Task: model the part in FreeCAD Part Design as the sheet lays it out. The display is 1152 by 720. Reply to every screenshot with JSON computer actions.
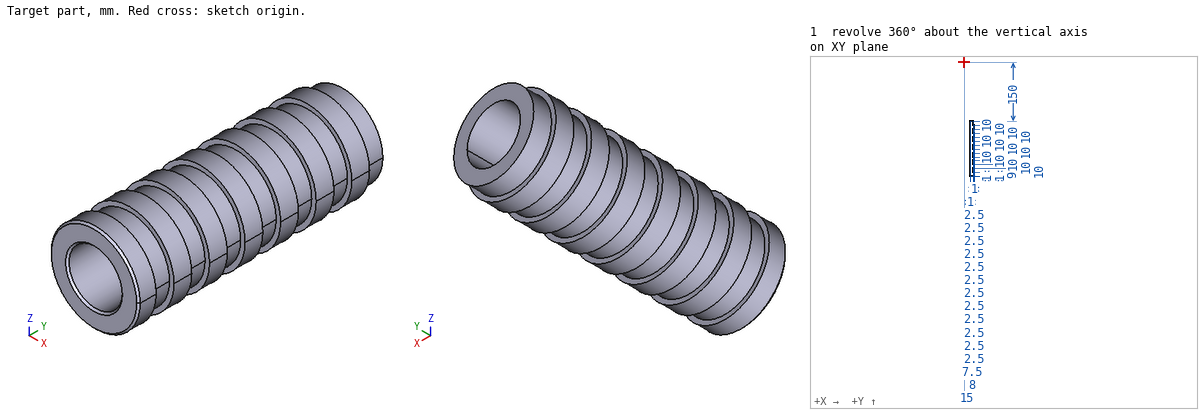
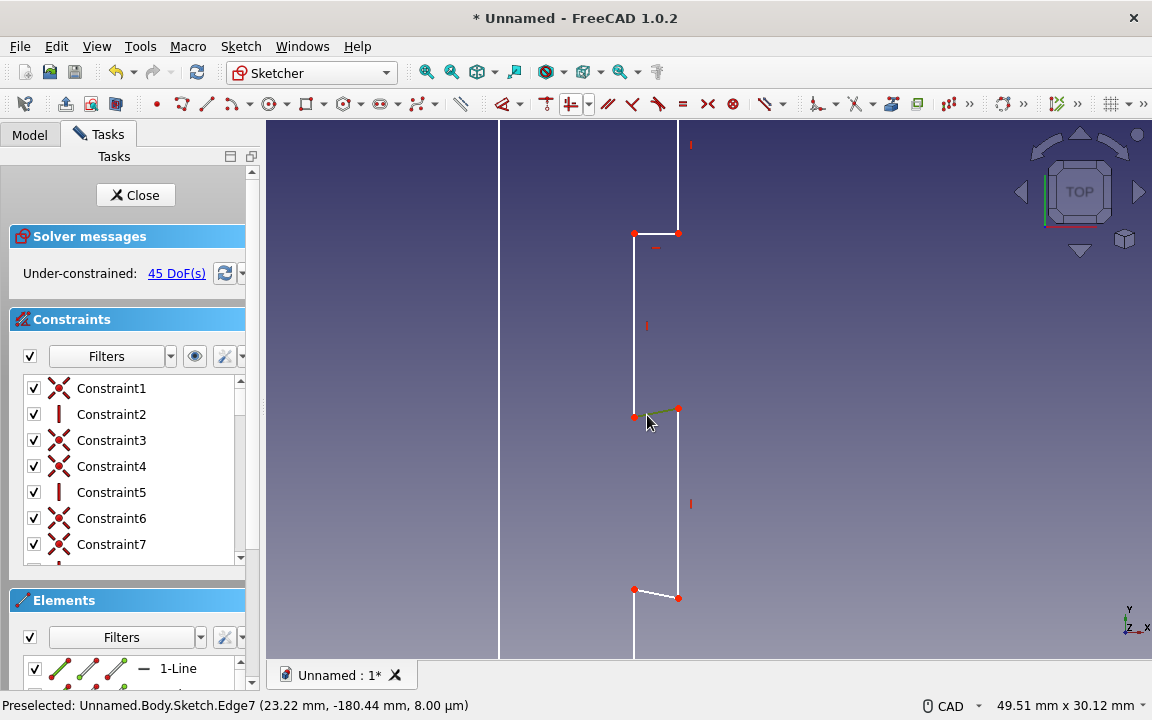
{"action": "key", "text": "h"}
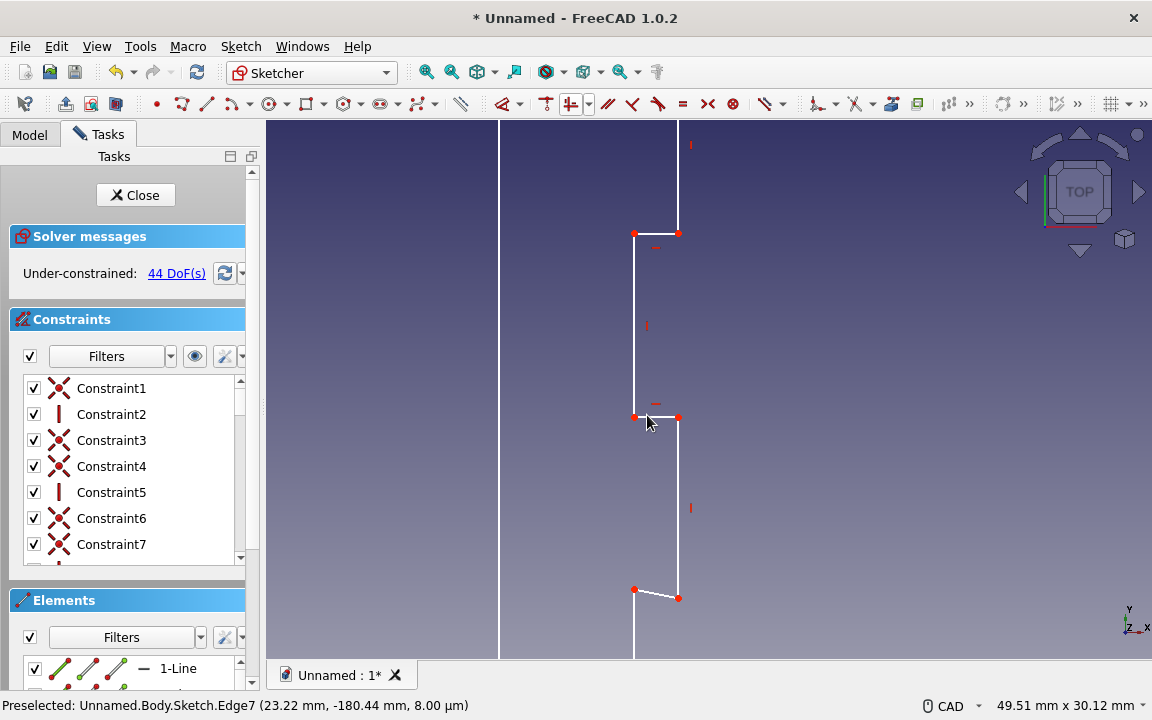
{"action": "left_click", "coordinate": [665, 596]}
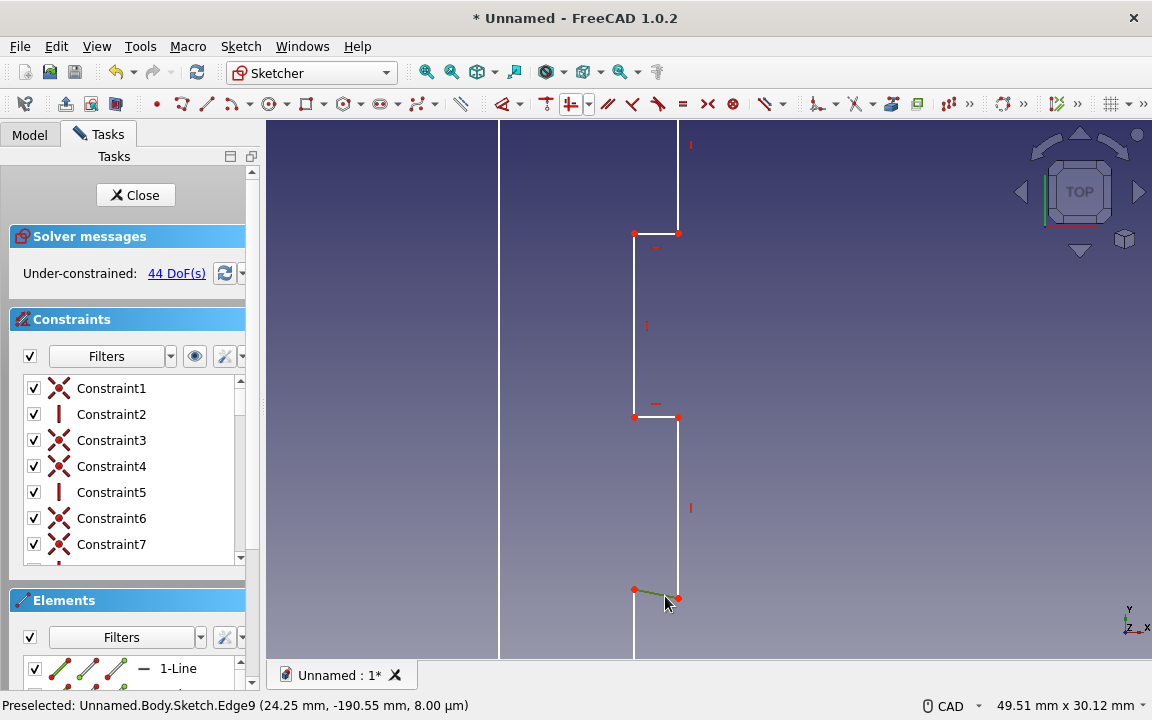
{"action": "left_click", "coordinate": [588, 104]}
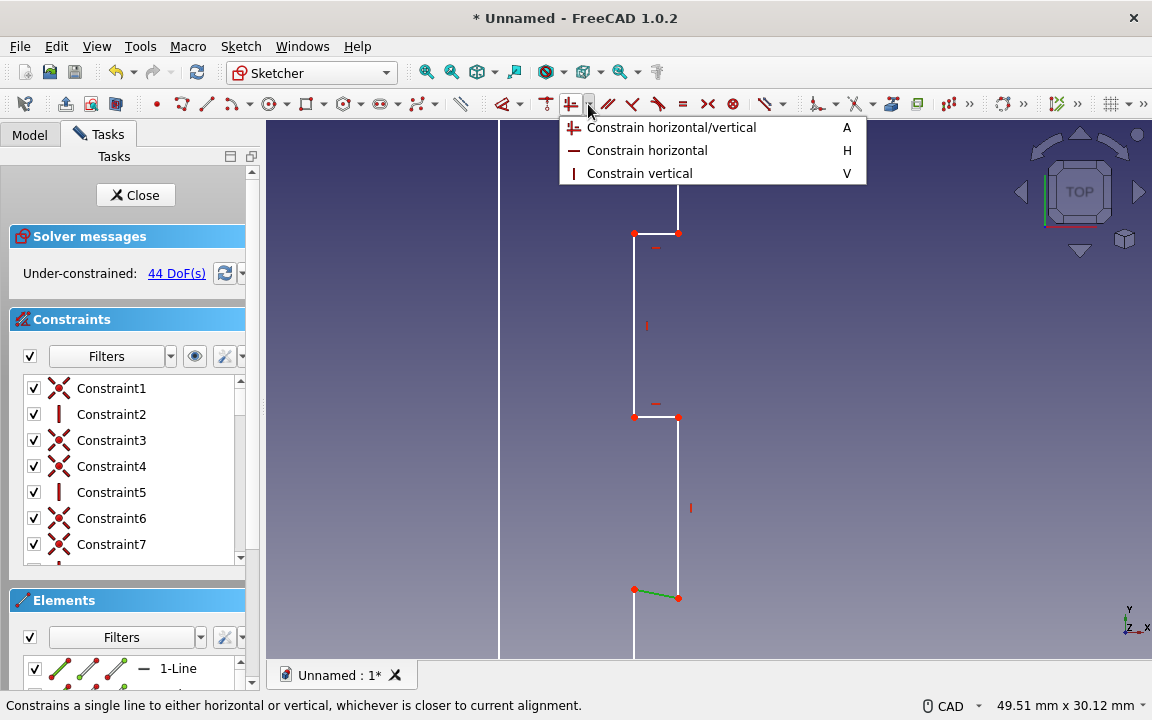
{"action": "left_click", "coordinate": [713, 150]}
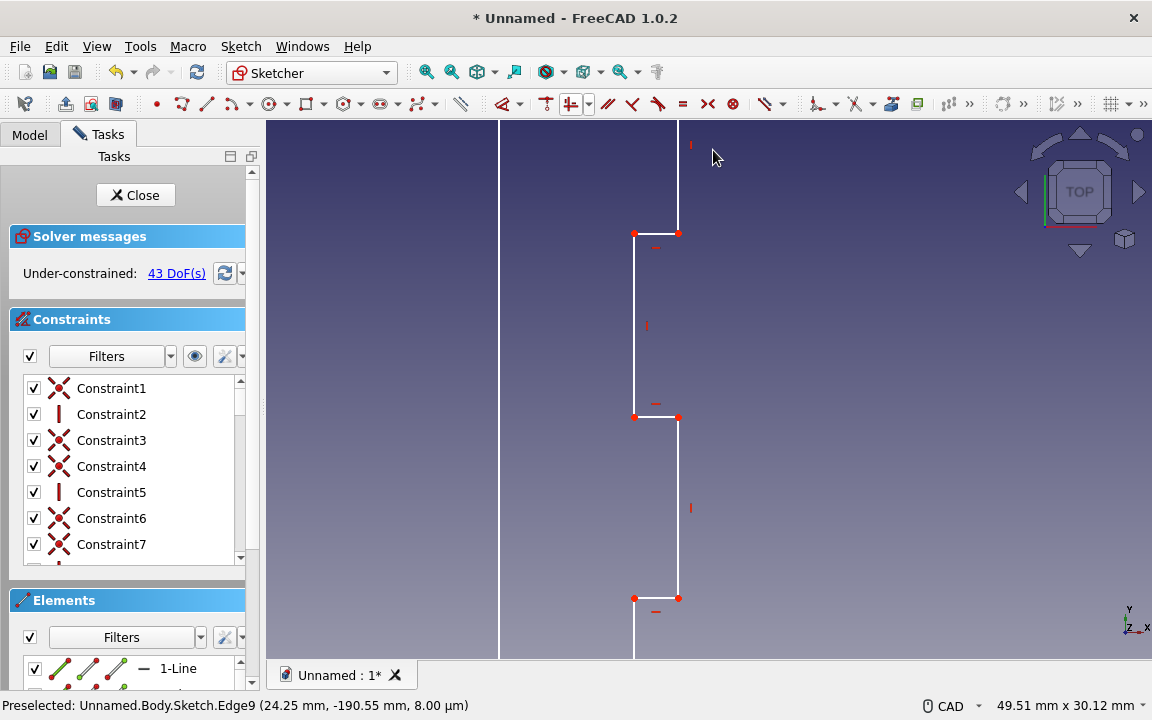
{"action": "scroll", "coordinate": [653, 429], "scroll_direction": "down", "scroll_amount": 14}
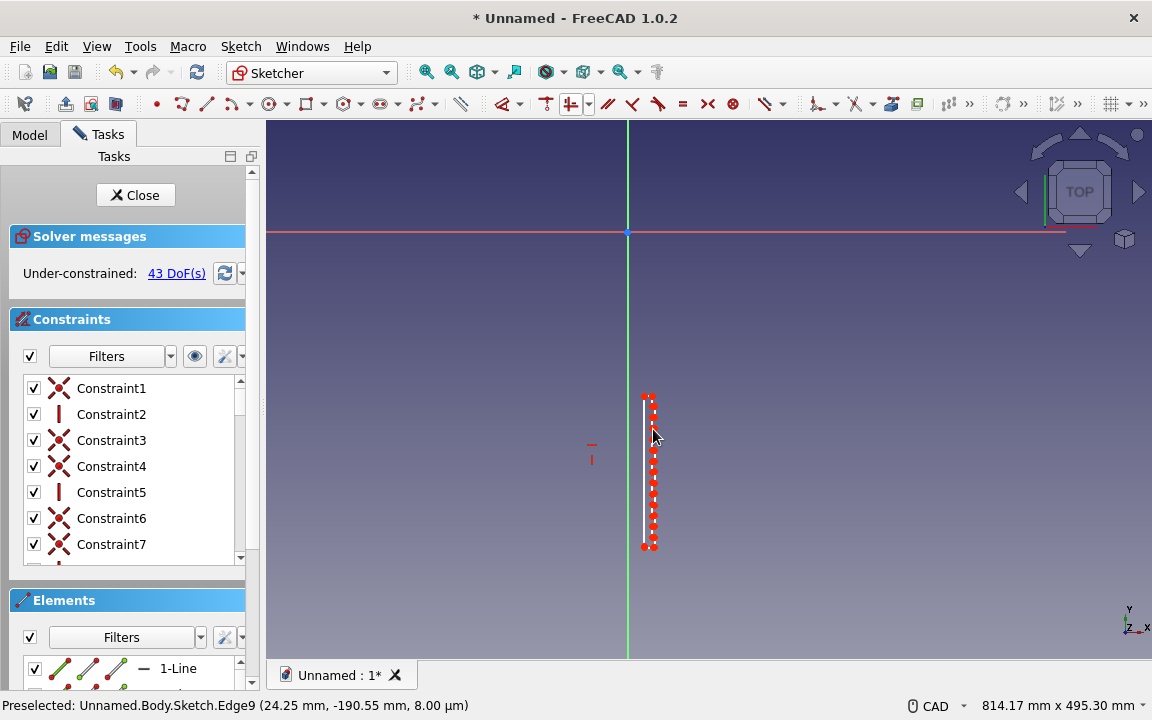
{"action": "scroll", "coordinate": [653, 451], "scroll_direction": "up", "scroll_amount": 14}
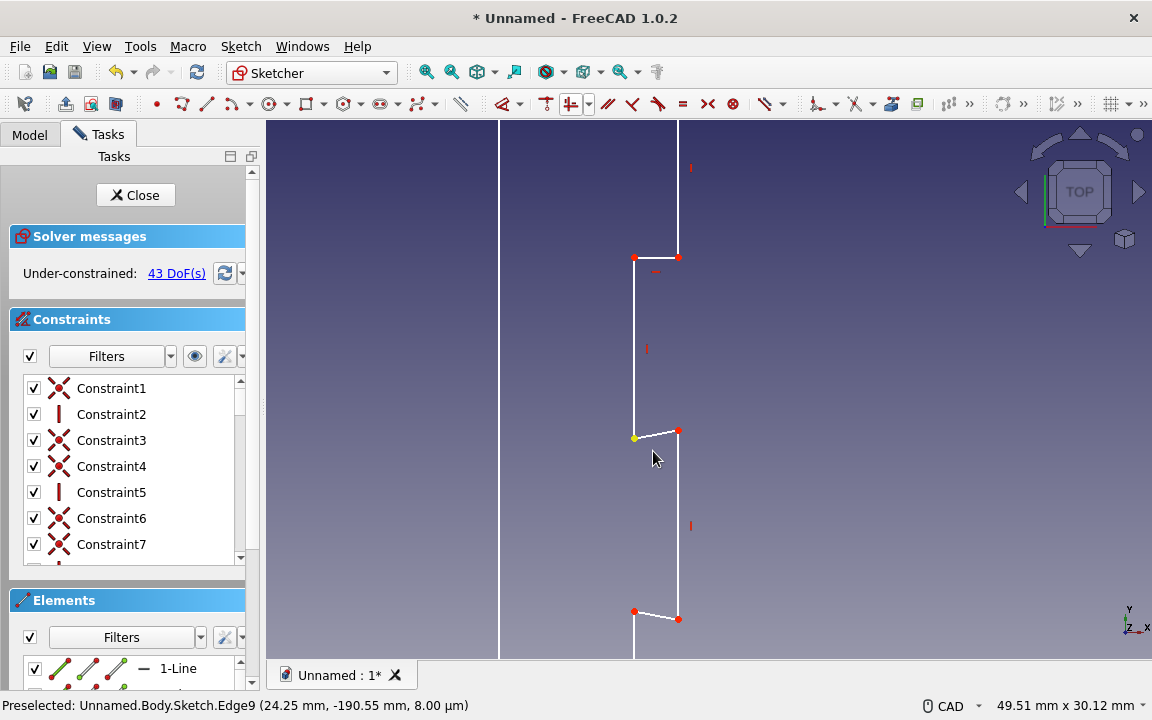
{"action": "left_click", "coordinate": [647, 436]}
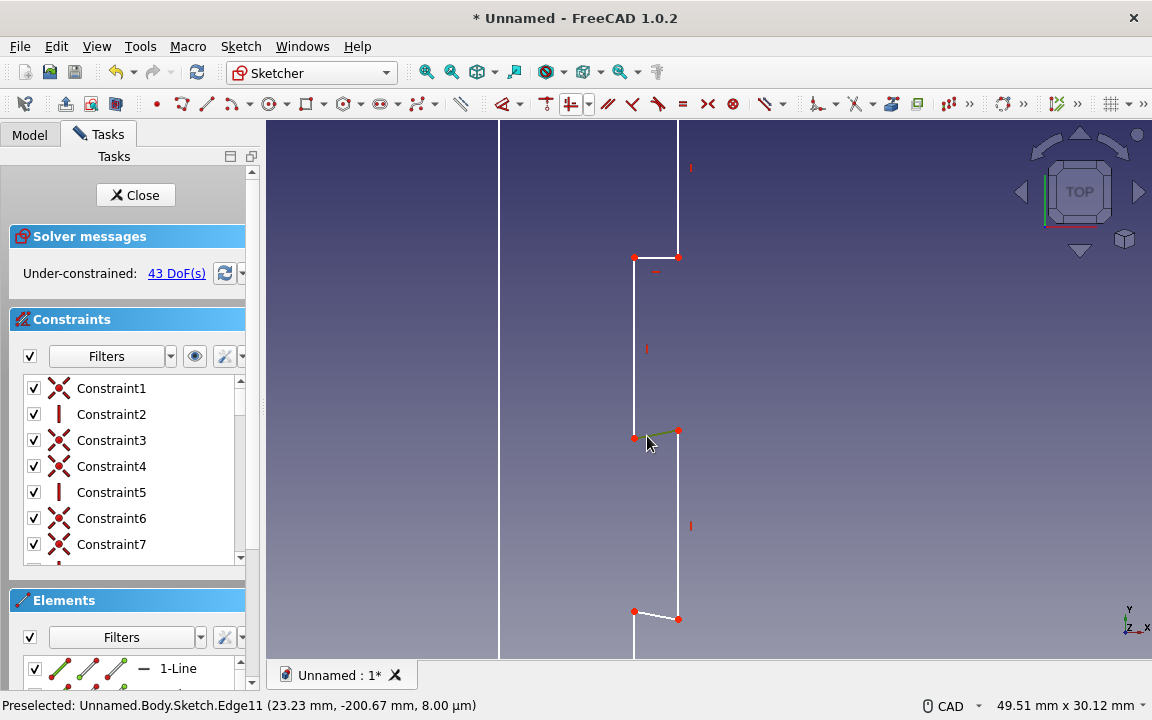
{"action": "key", "text": "h"}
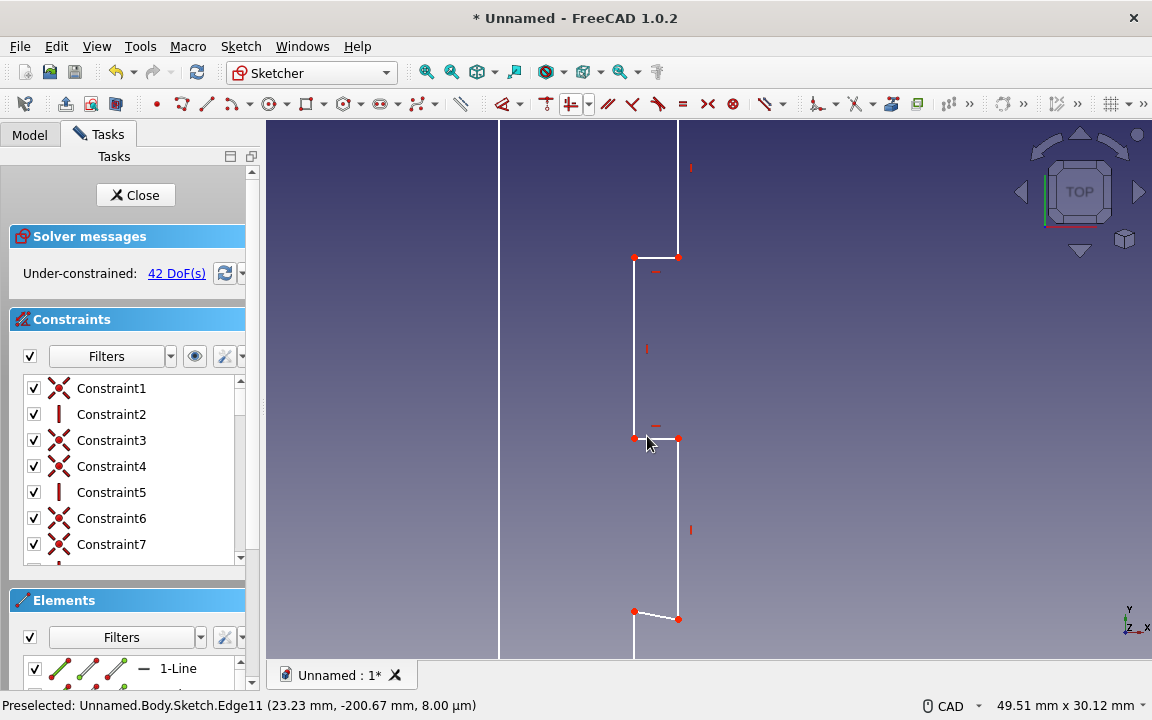
{"action": "left_click", "coordinate": [665, 617]}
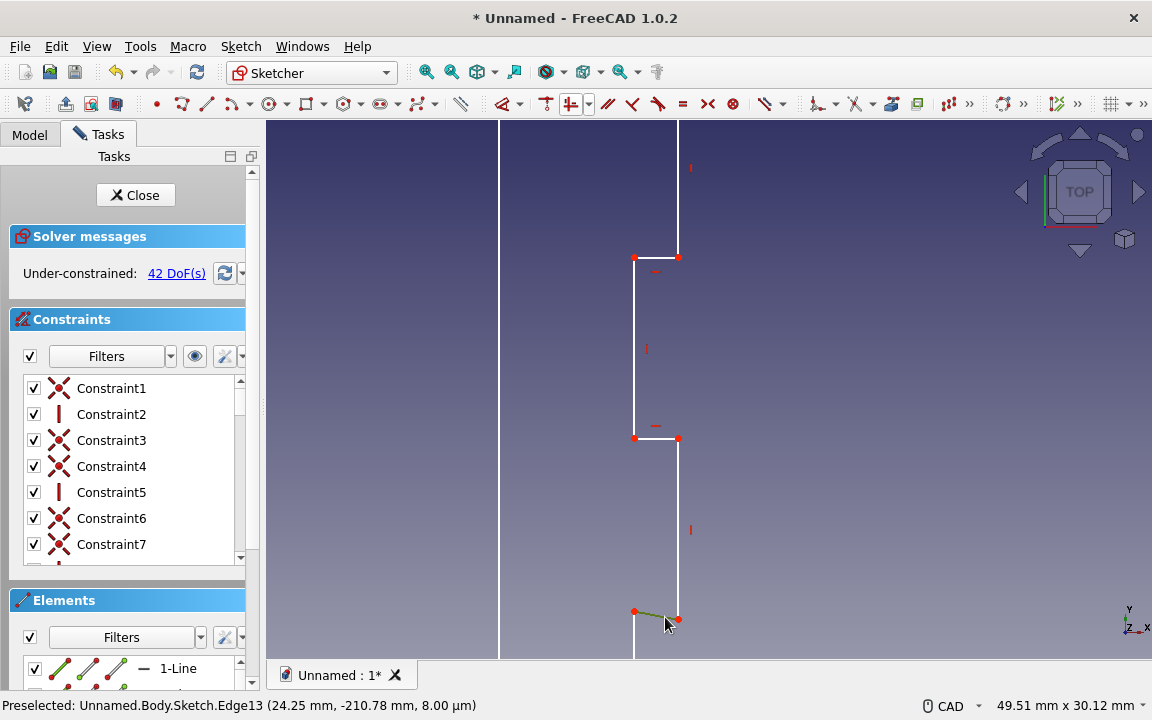
{"action": "key", "text": "h"}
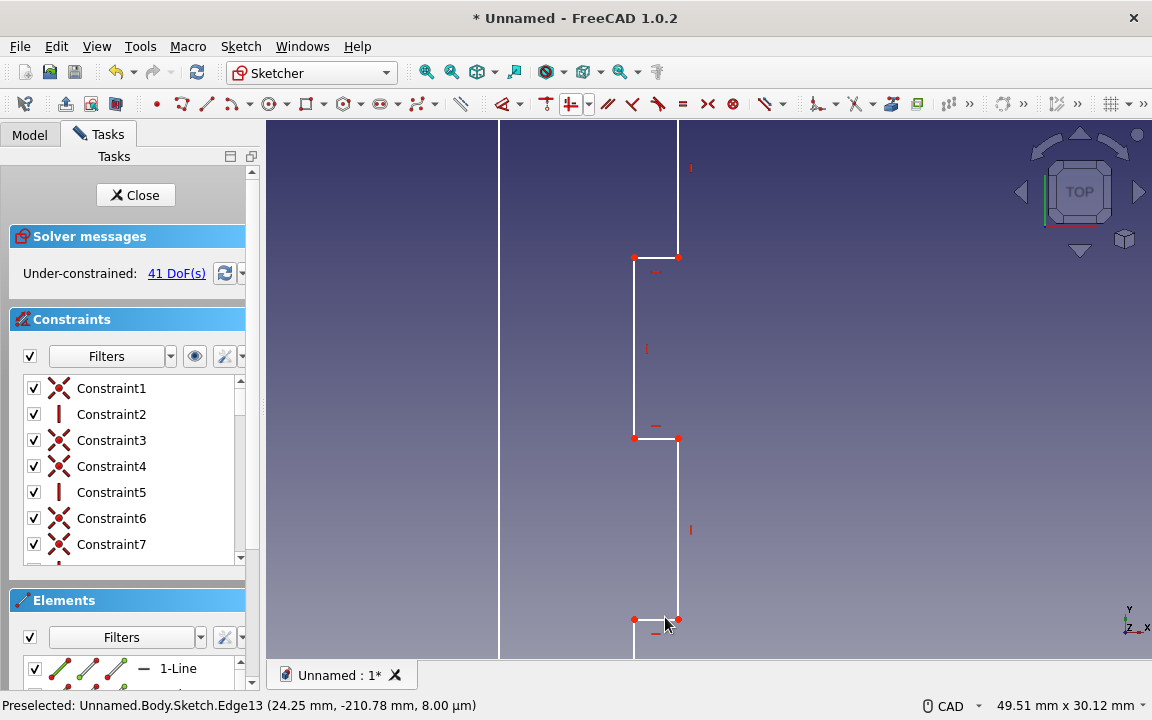
{"action": "scroll", "coordinate": [653, 451], "scroll_direction": "down", "scroll_amount": 14}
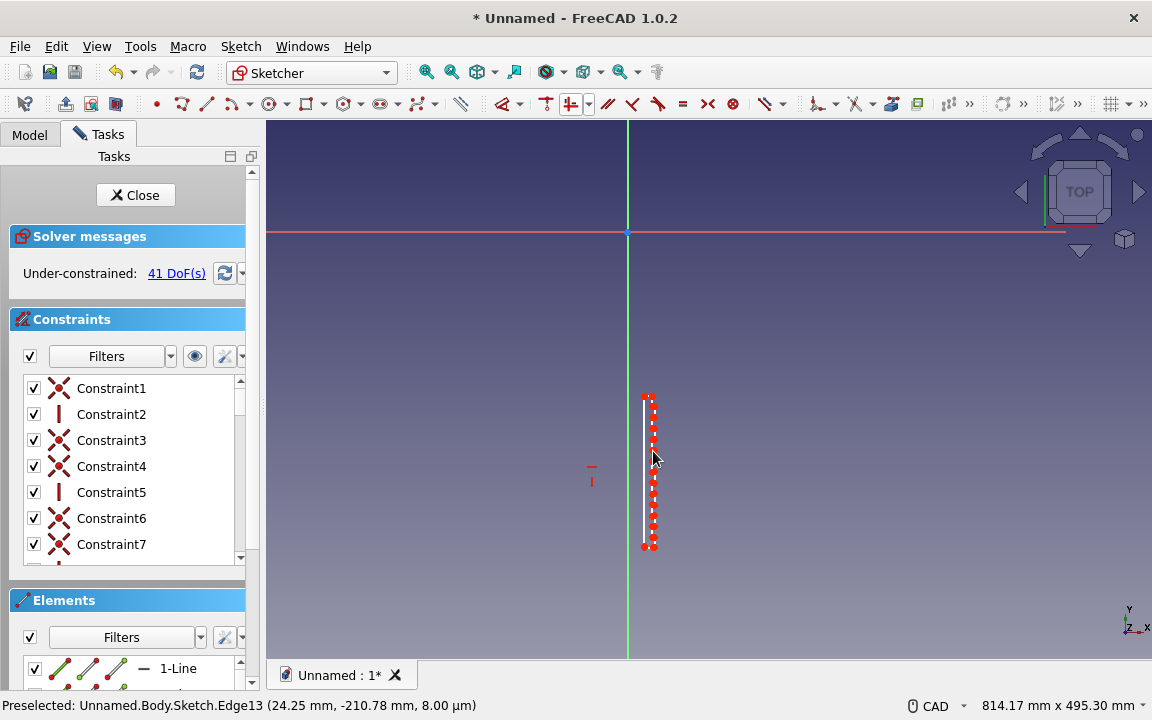
{"action": "scroll", "coordinate": [653, 472], "scroll_direction": "up", "scroll_amount": 14}